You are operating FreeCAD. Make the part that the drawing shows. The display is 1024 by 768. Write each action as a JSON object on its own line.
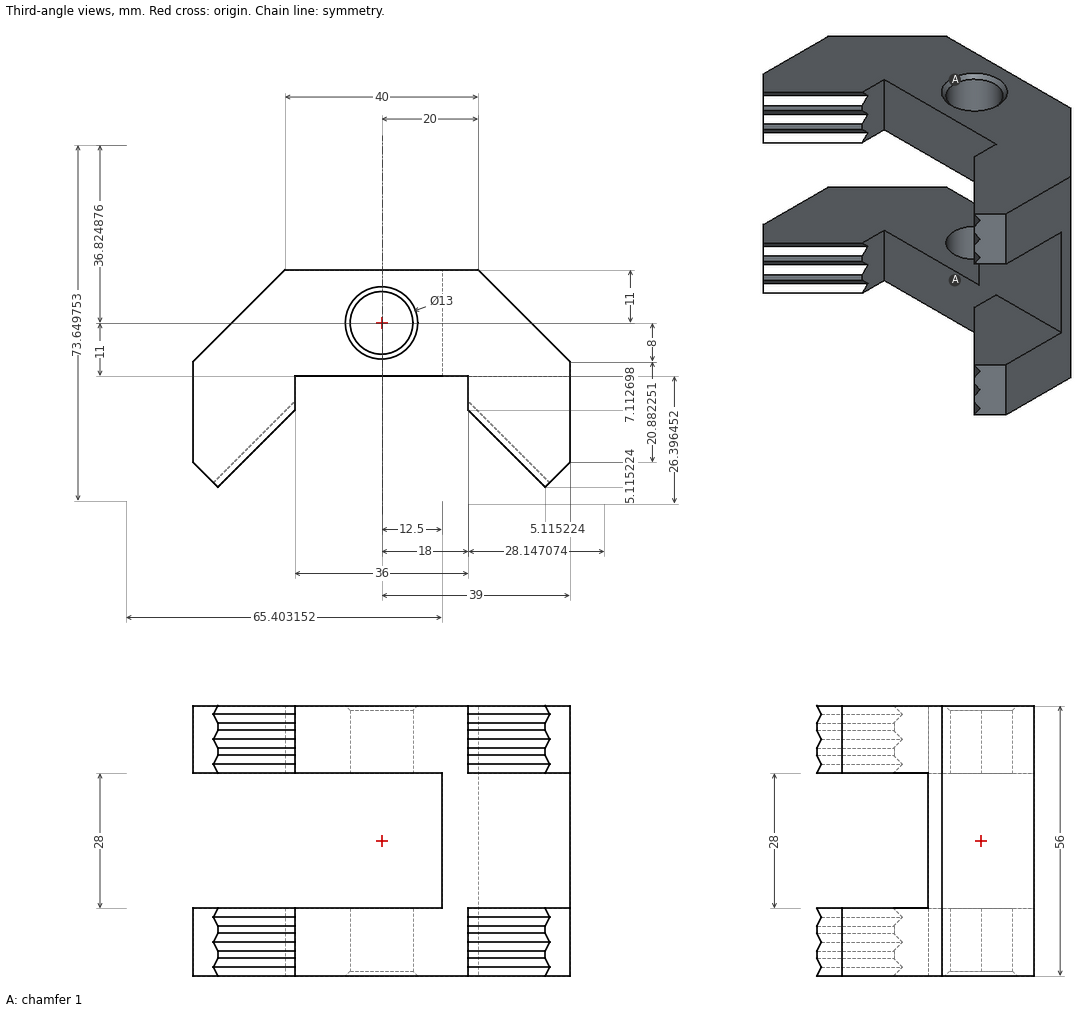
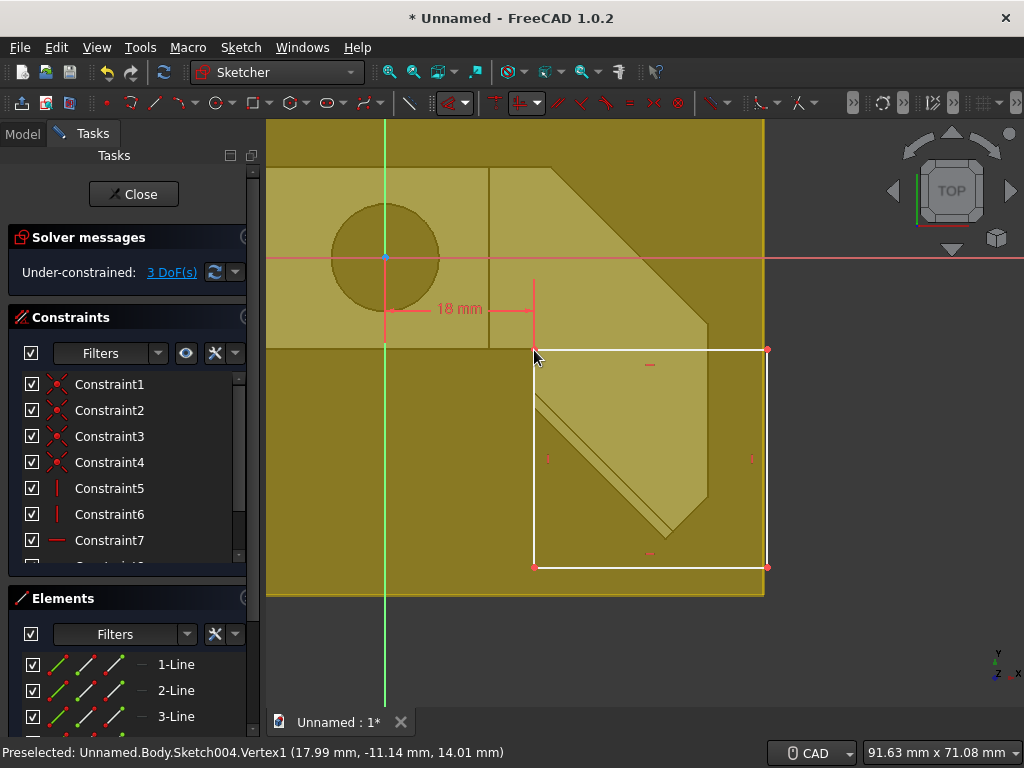
{"action": "left_click", "coordinate": [534, 350]}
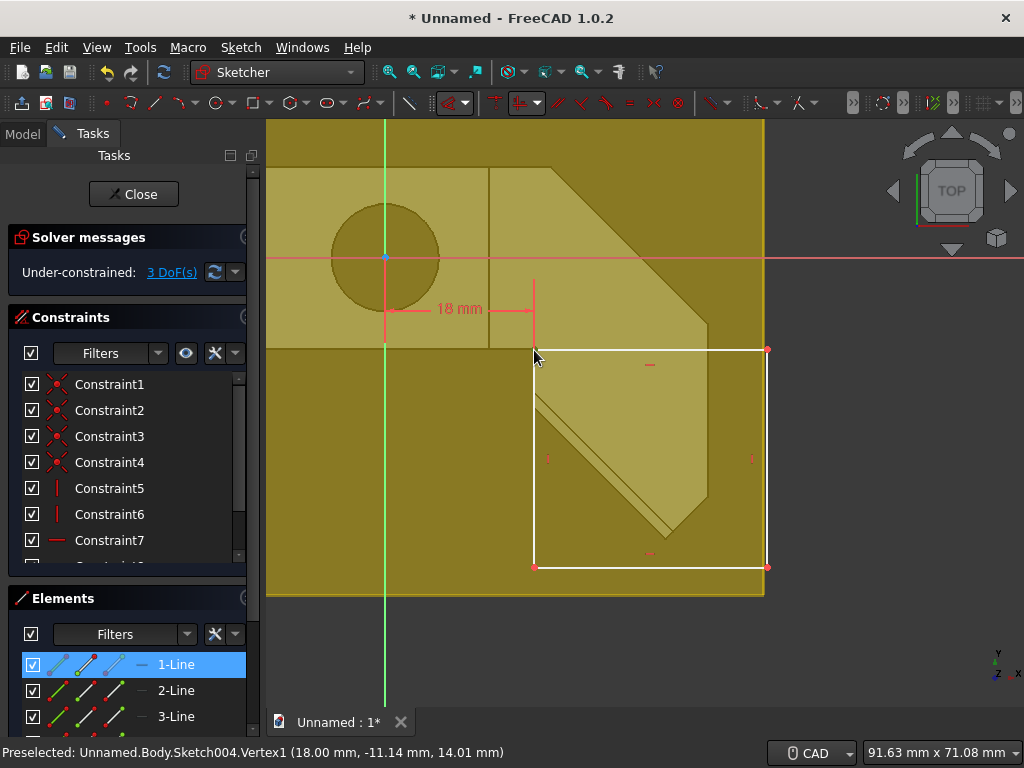
{"action": "left_click", "coordinate": [468, 104]}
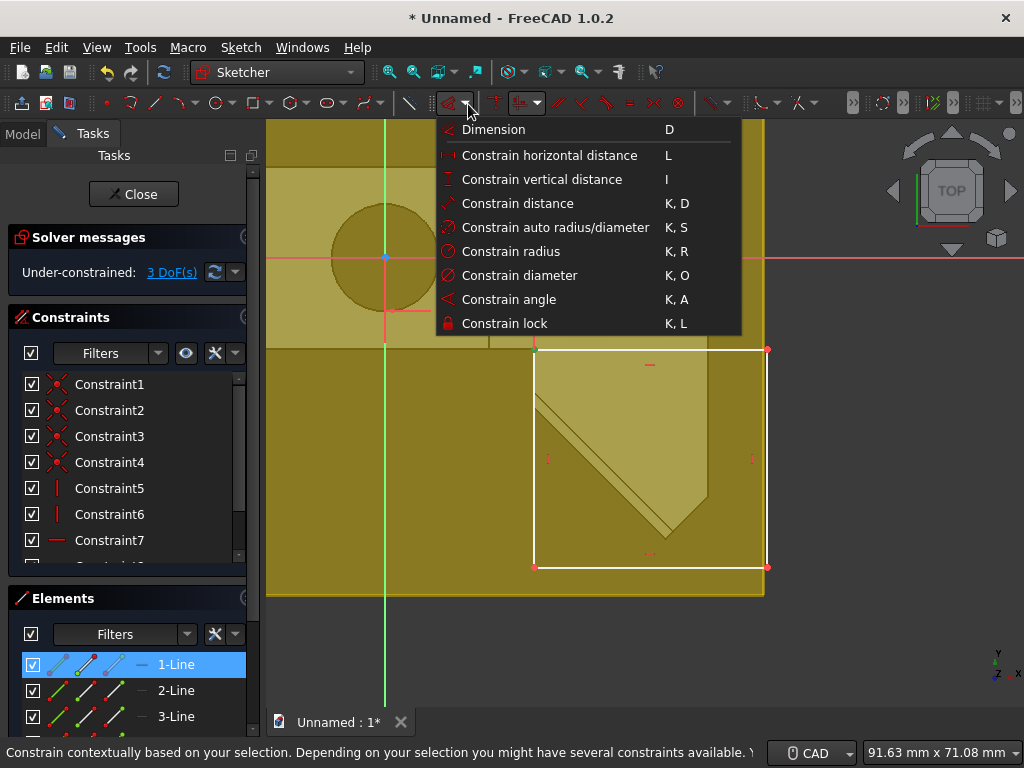
{"action": "left_click", "coordinate": [589, 179]}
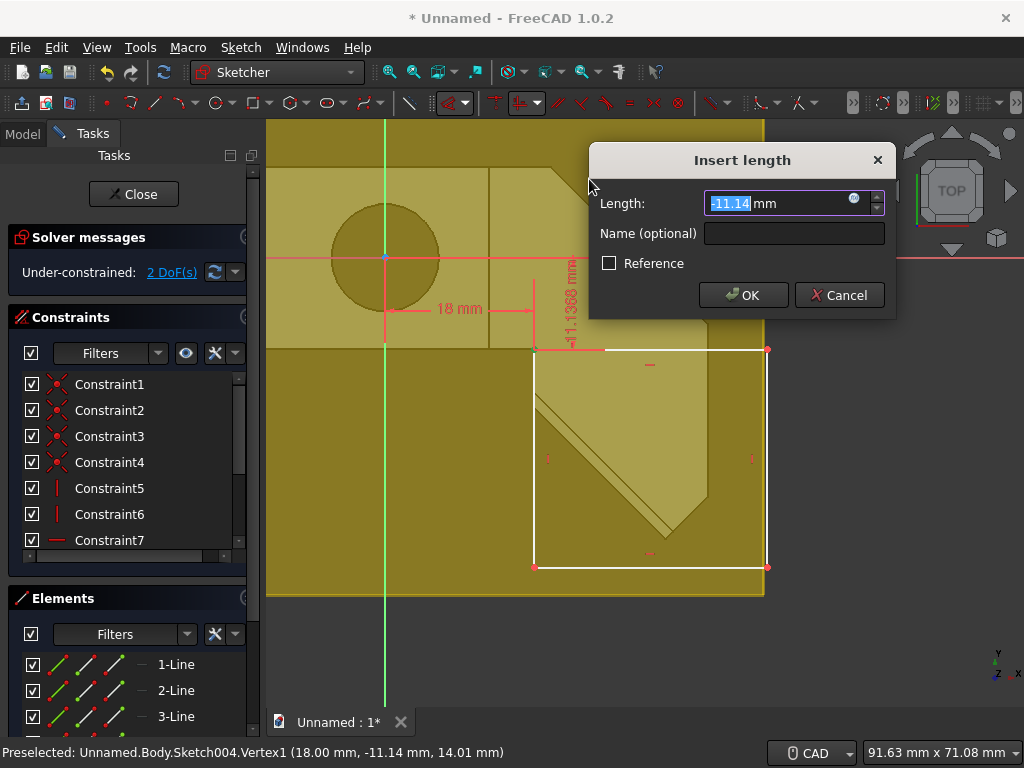
{"action": "type", "text": "-11"}
{"action": "key", "text": "Return"}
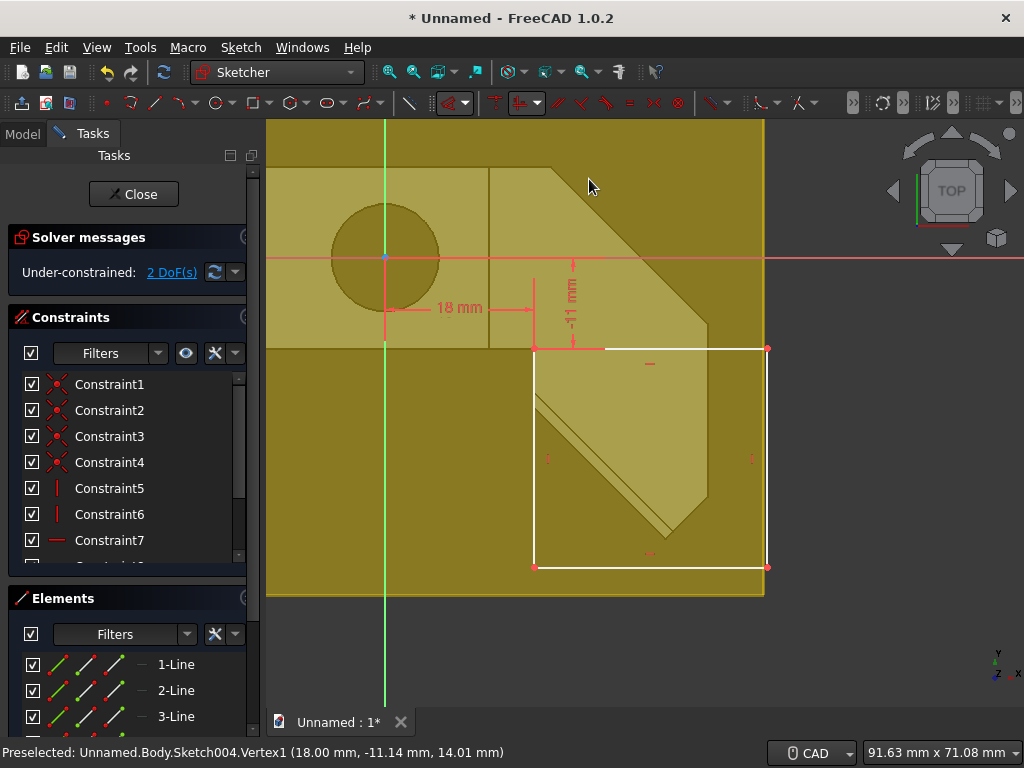
{"action": "left_click", "coordinate": [534, 415]}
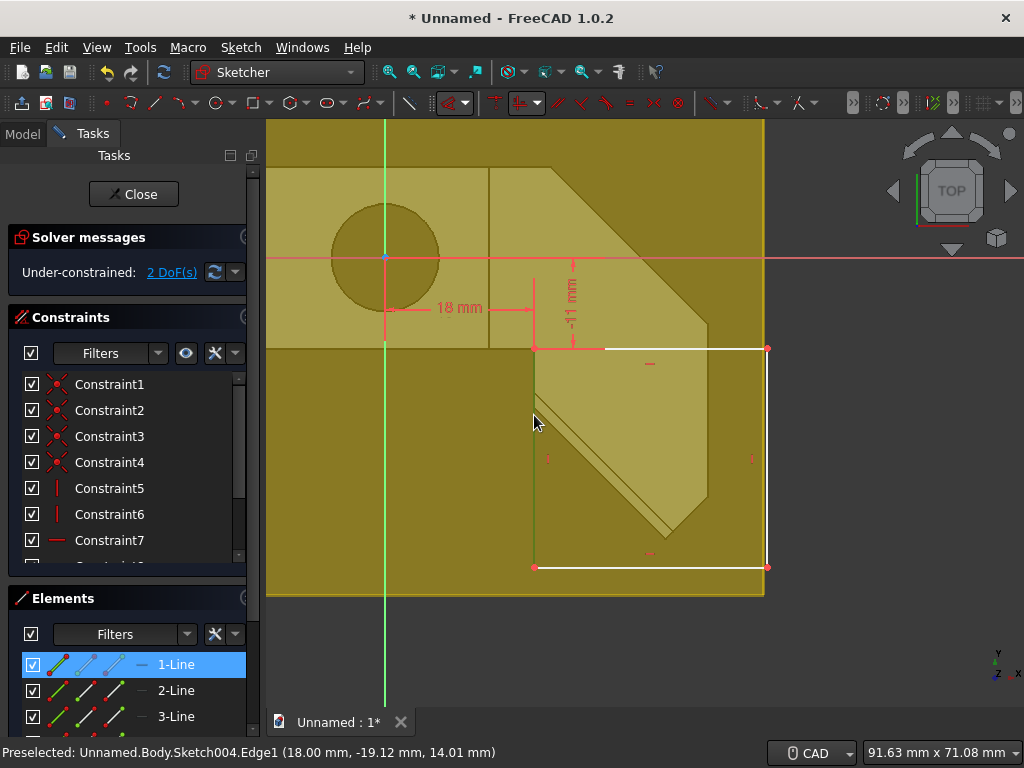
{"action": "key", "text": "i"}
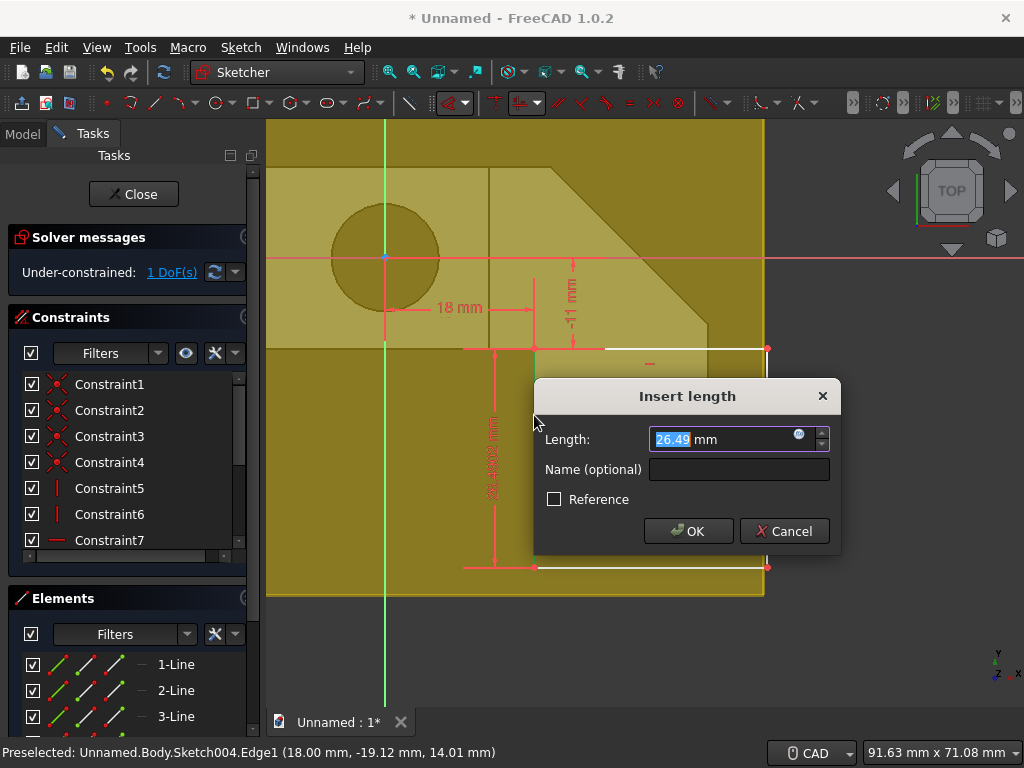
{"action": "type", "text": "26.396452"}
{"action": "key", "text": "Return"}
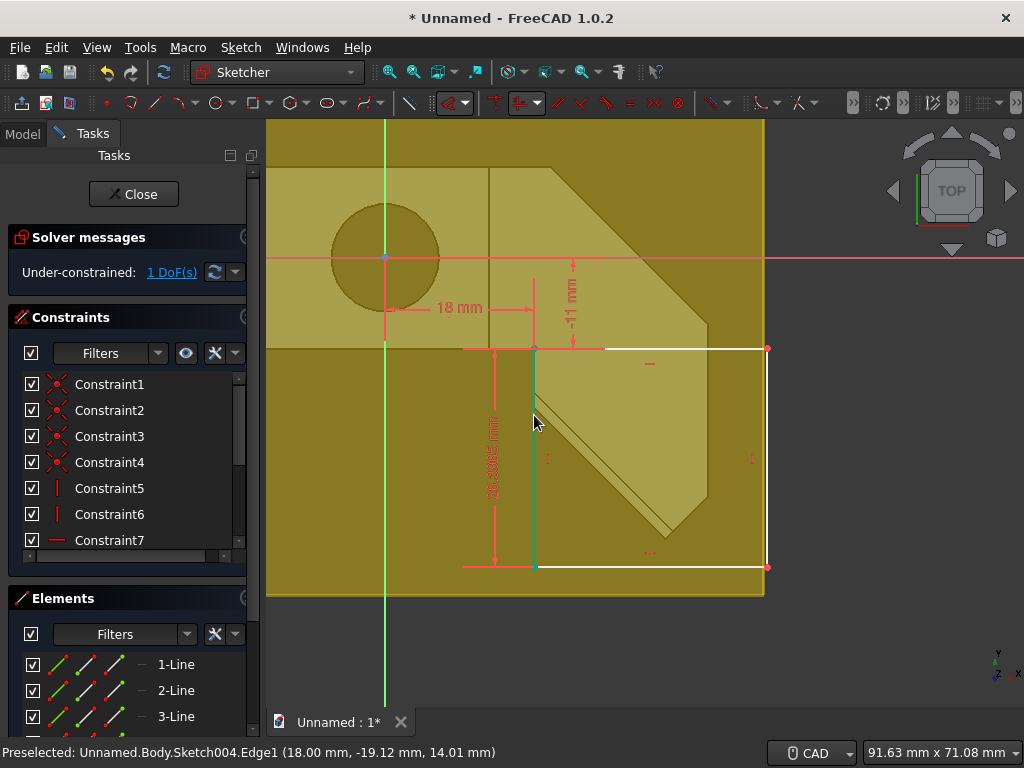
{"action": "left_click", "coordinate": [604, 567]}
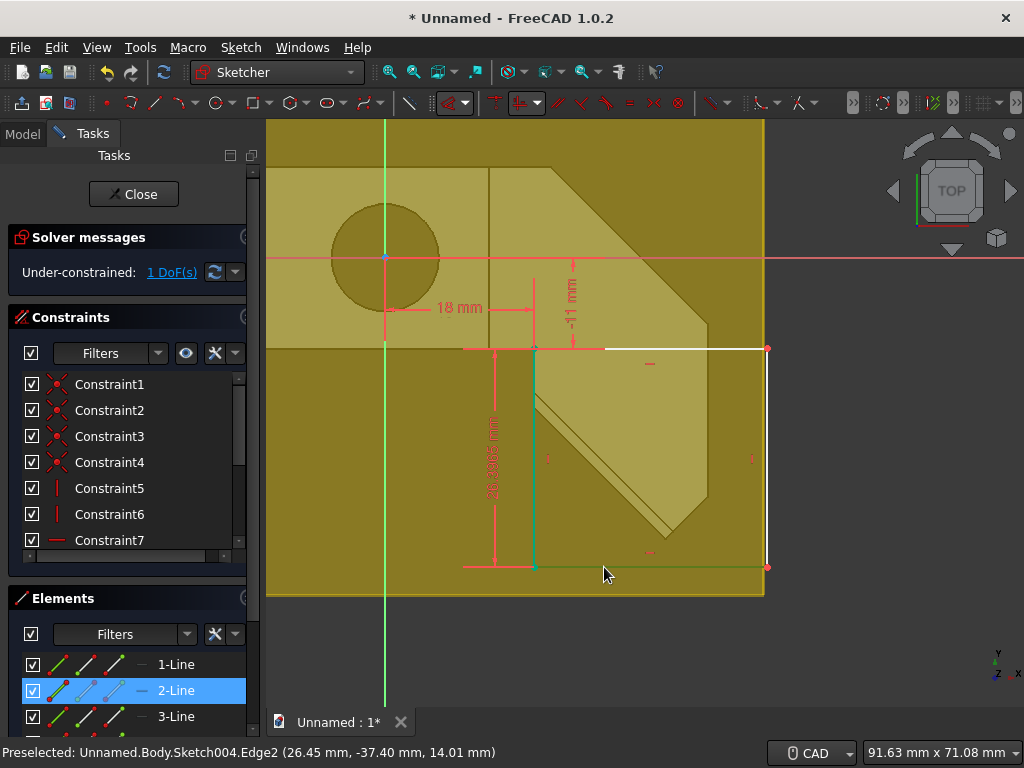
{"action": "key", "text": "l"}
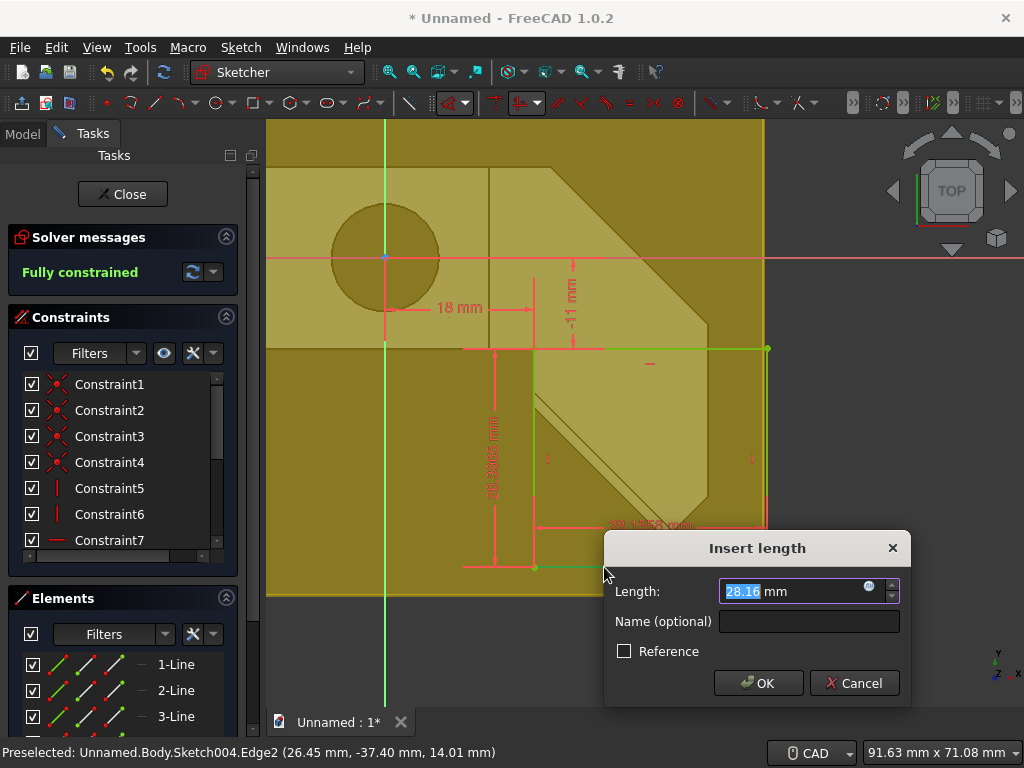
{"action": "type", "text": "28.147074"}
{"action": "key", "text": "Return"}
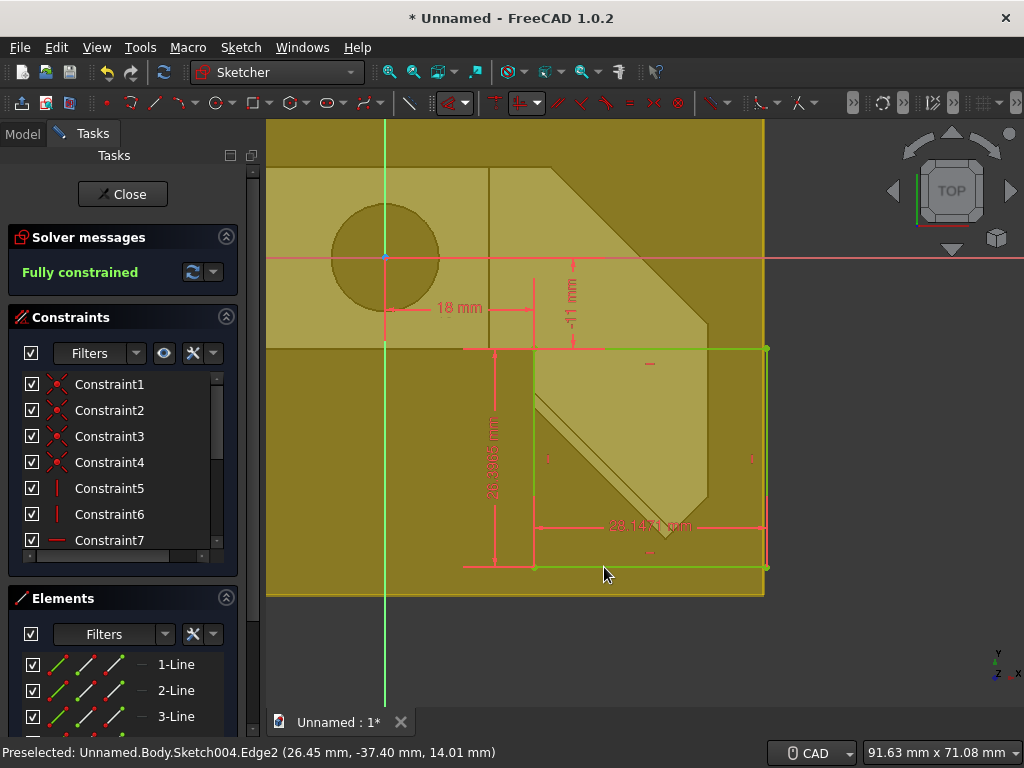
{"action": "left_click", "coordinate": [123, 194]}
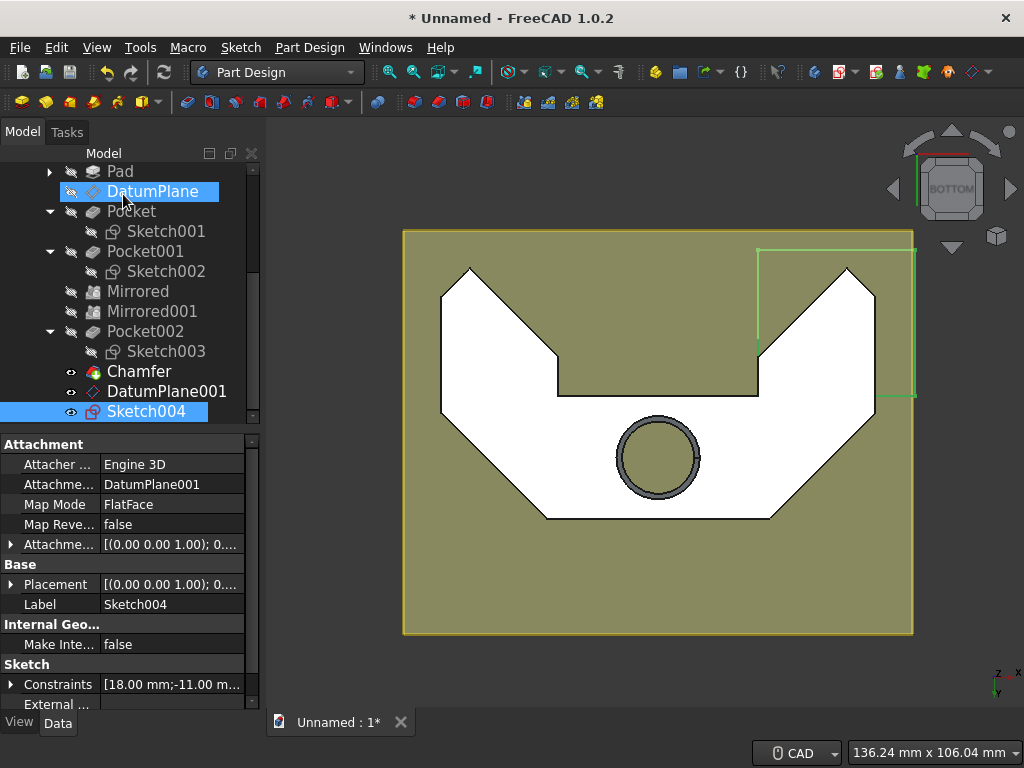
{"action": "left_click", "coordinate": [188, 102]}